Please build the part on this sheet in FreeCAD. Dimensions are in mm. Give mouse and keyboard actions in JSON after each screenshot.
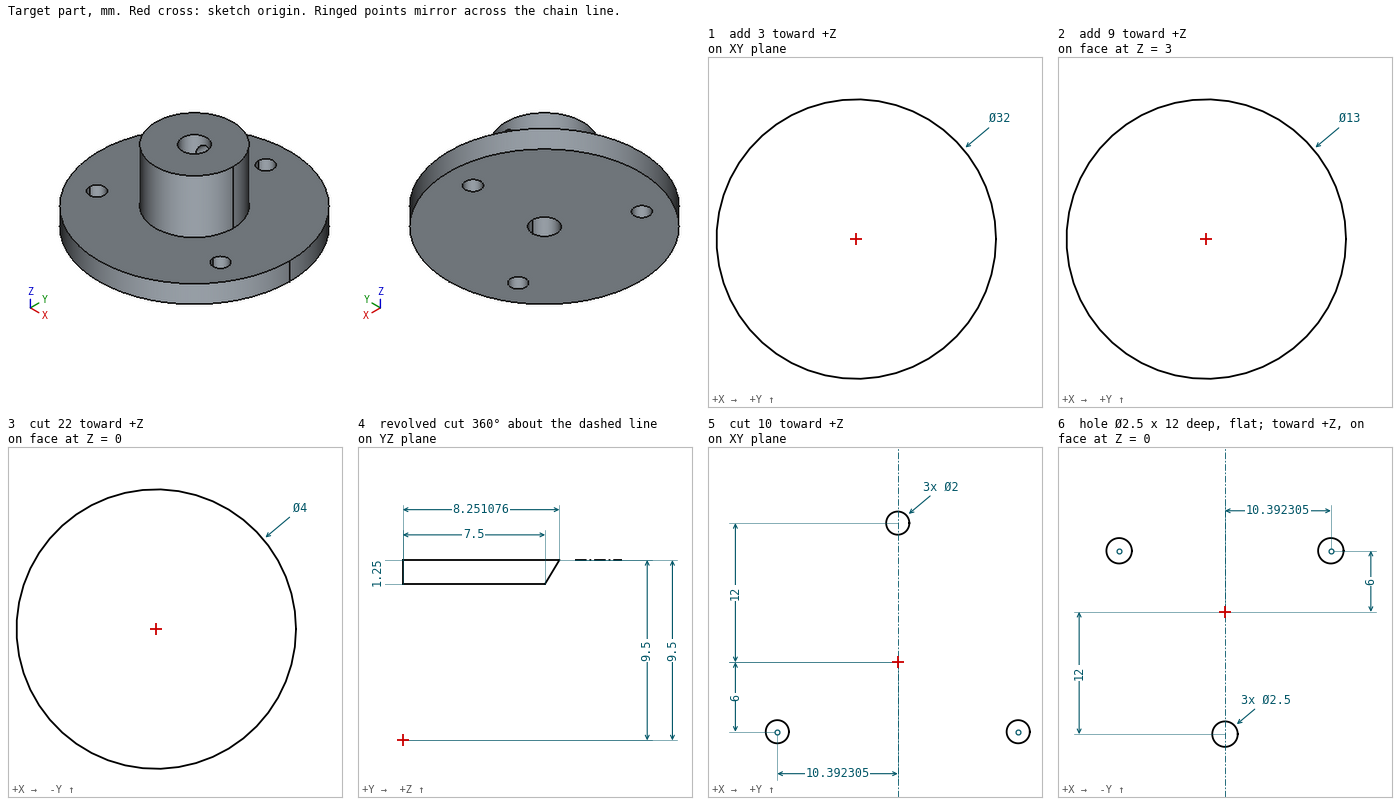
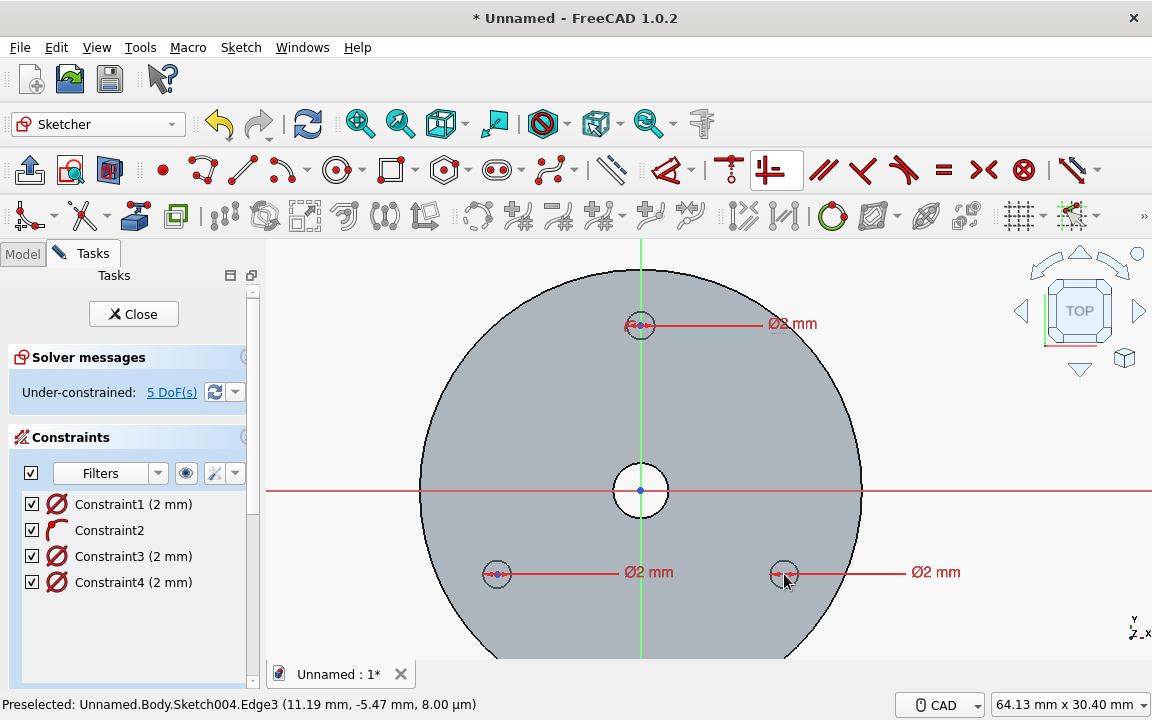
{"action": "left_click", "coordinate": [497, 574]}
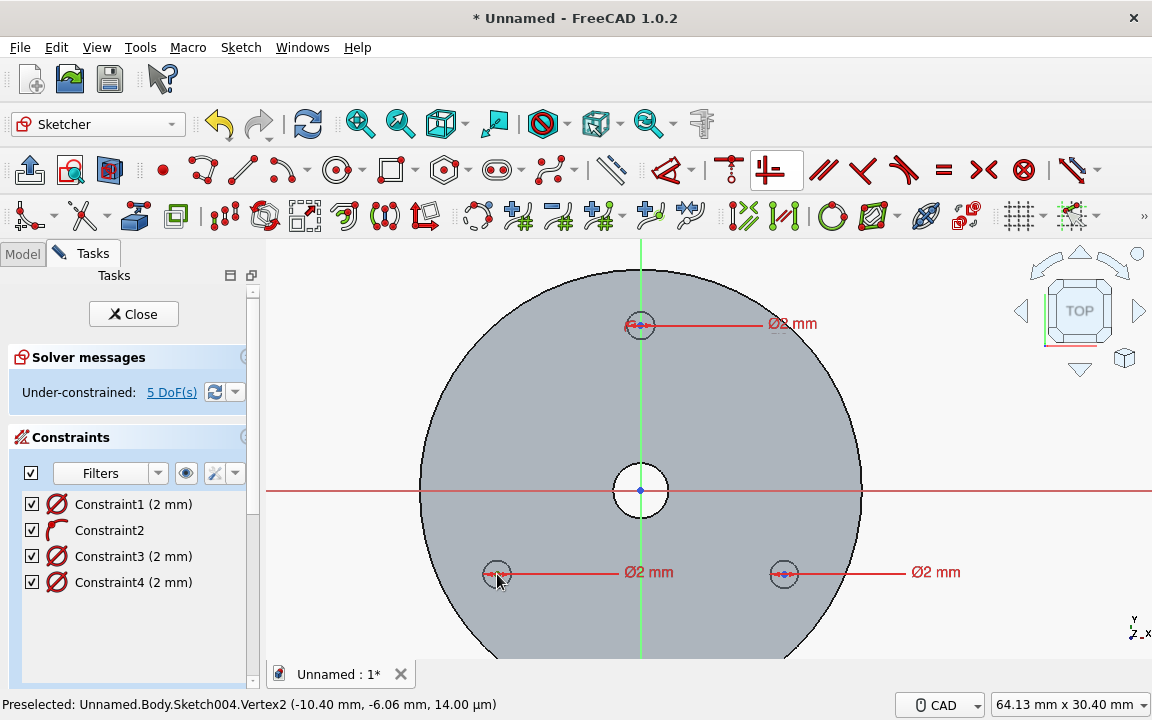
{"action": "left_click", "coordinate": [784, 574]}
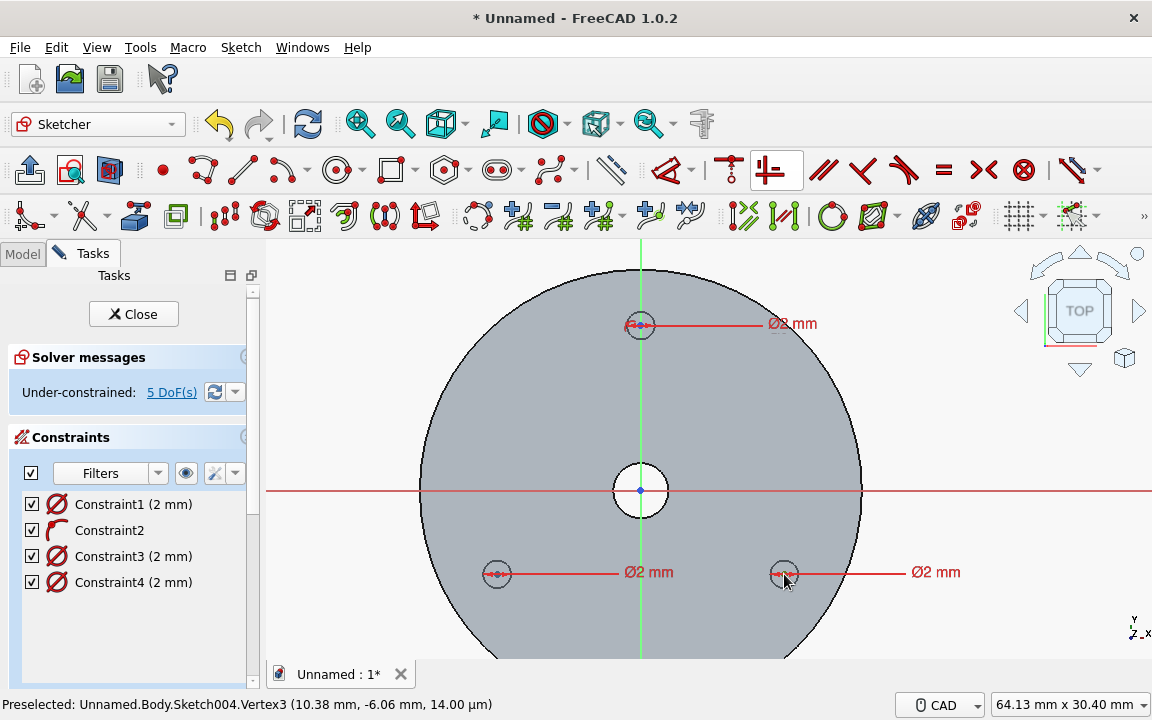
{"action": "left_click", "coordinate": [641, 605]}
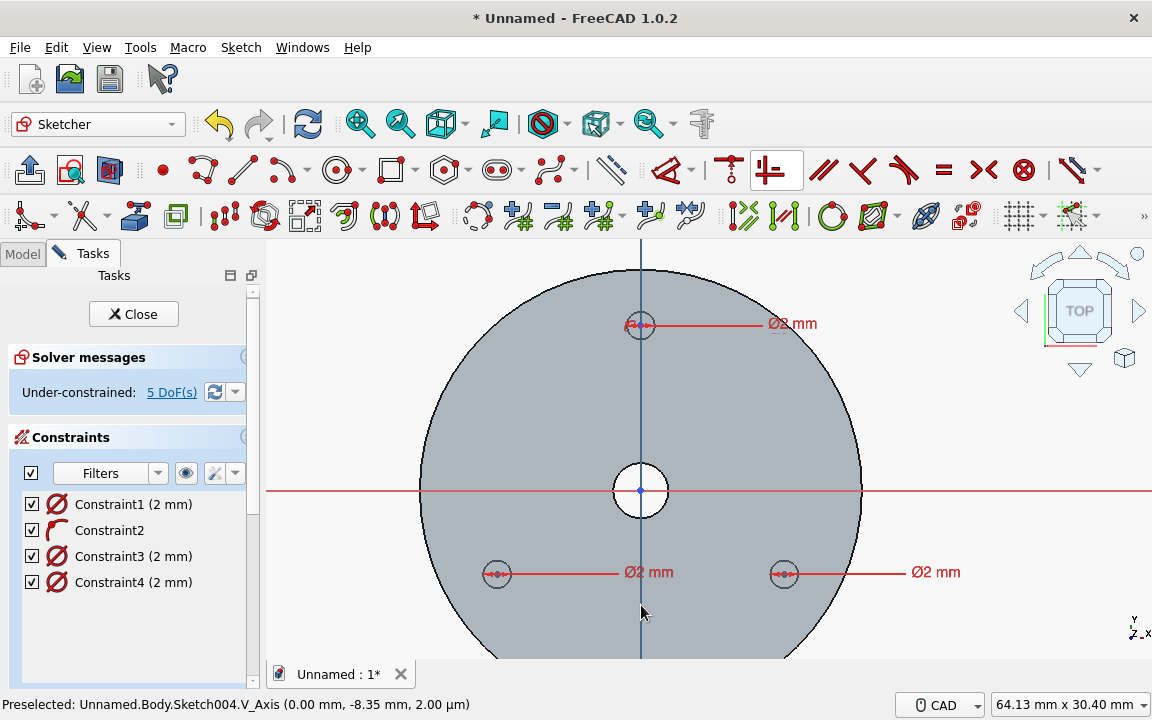
{"action": "left_click", "coordinate": [984, 170]}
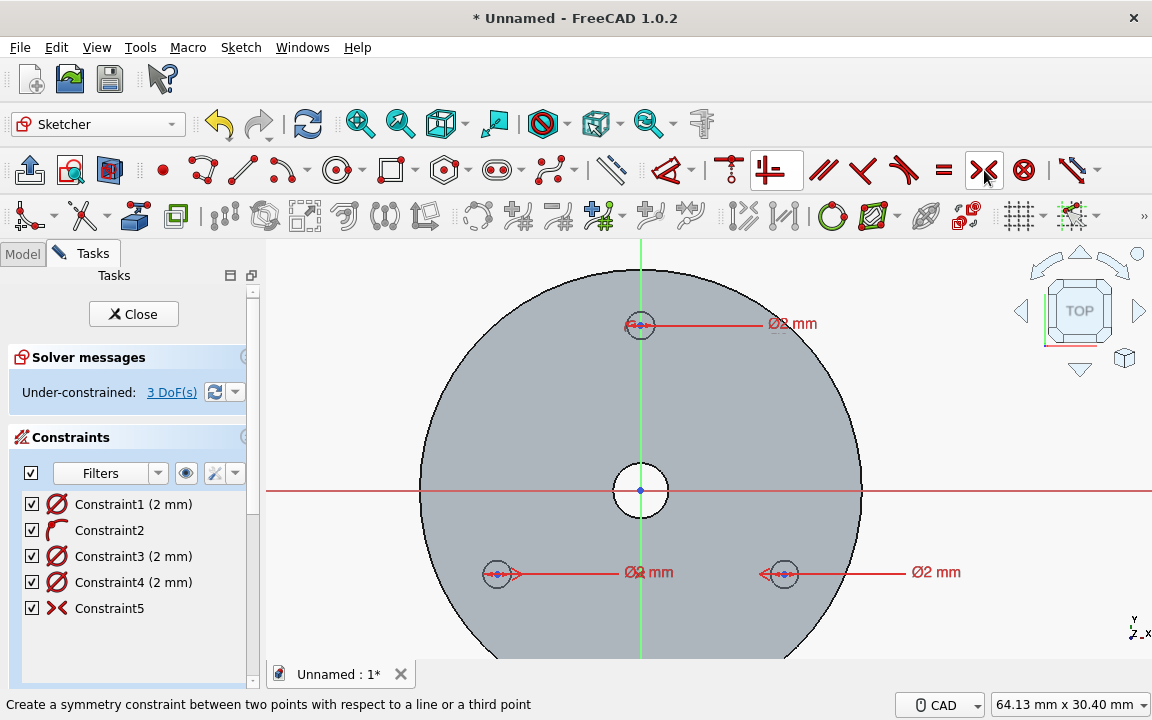
{"action": "left_click", "coordinate": [666, 170]}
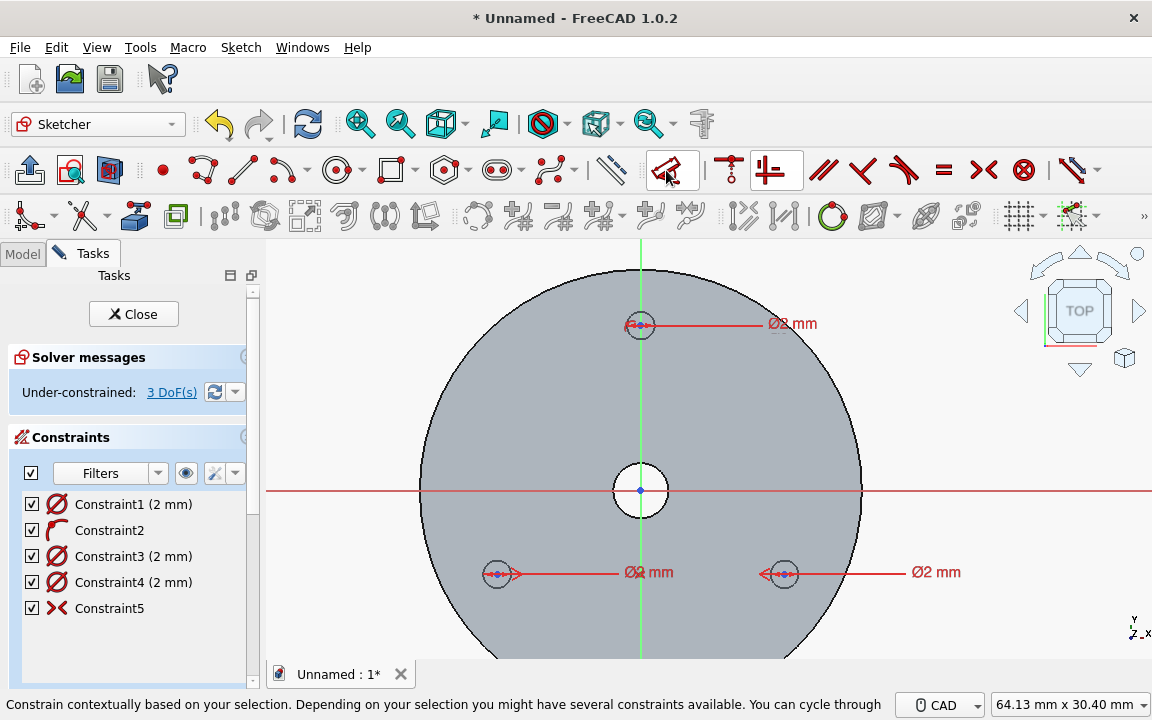
{"action": "left_click", "coordinate": [497, 574]}
{"action": "left_click", "coordinate": [463, 533]}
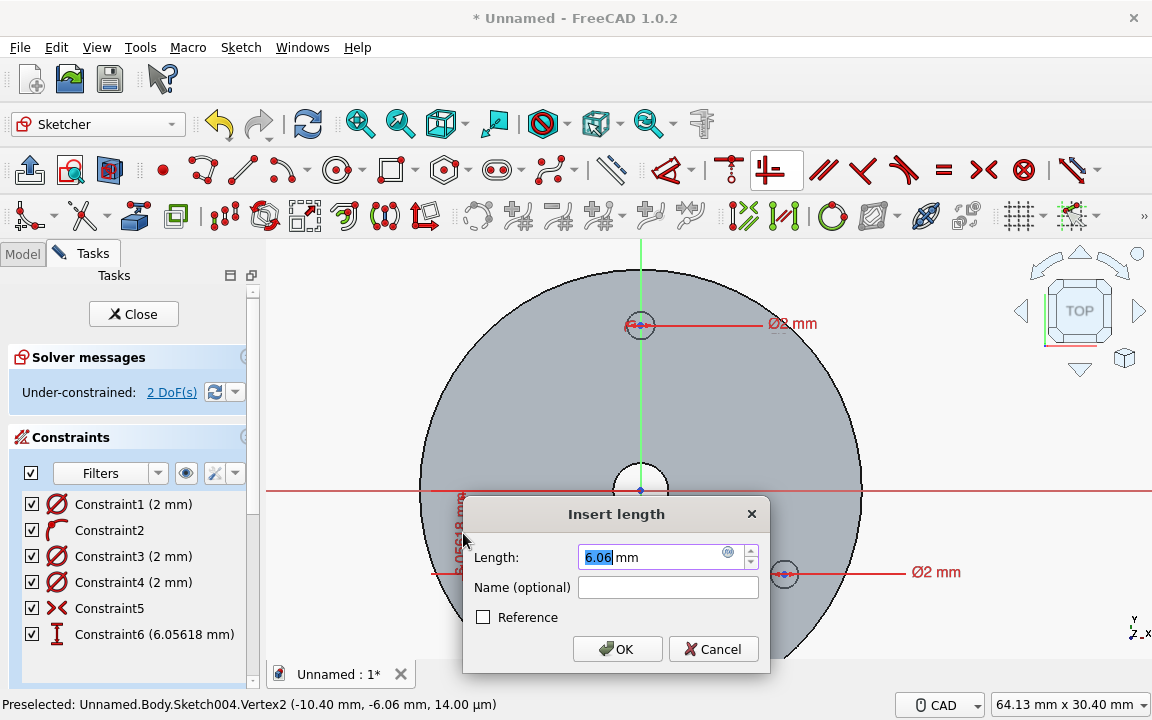
{"action": "type", "text": "6"}
{"action": "key", "text": "Return"}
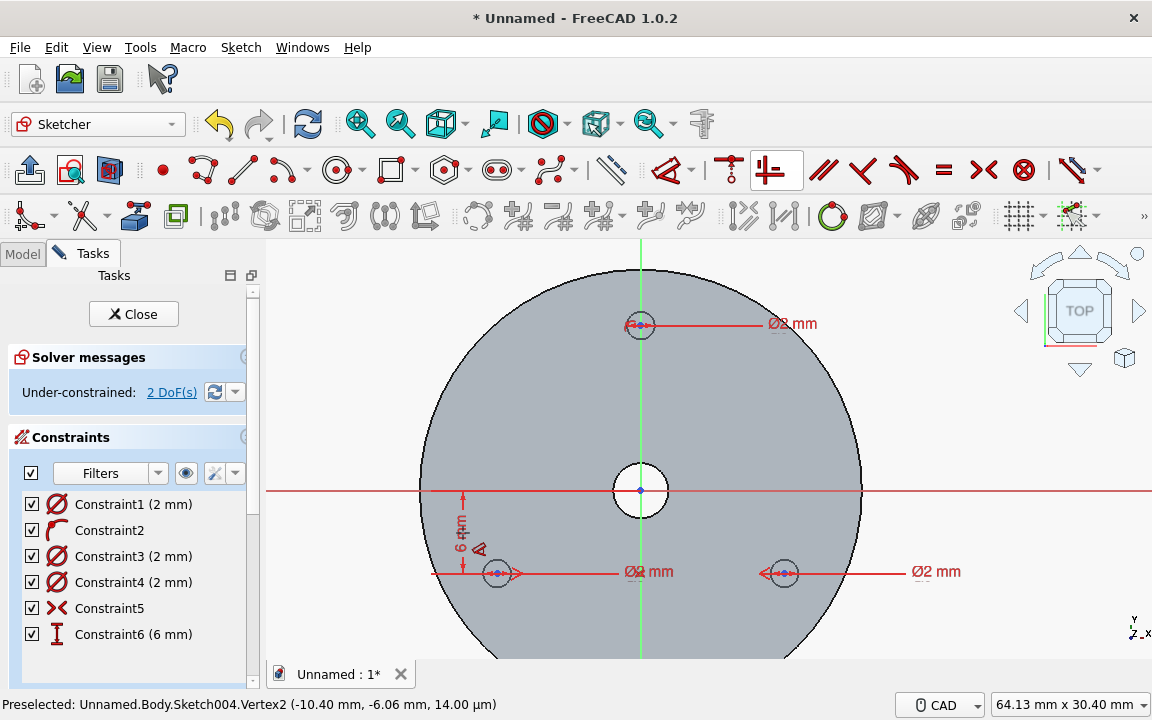
{"action": "left_click", "coordinate": [641, 326]}
{"action": "left_click", "coordinate": [675, 408]}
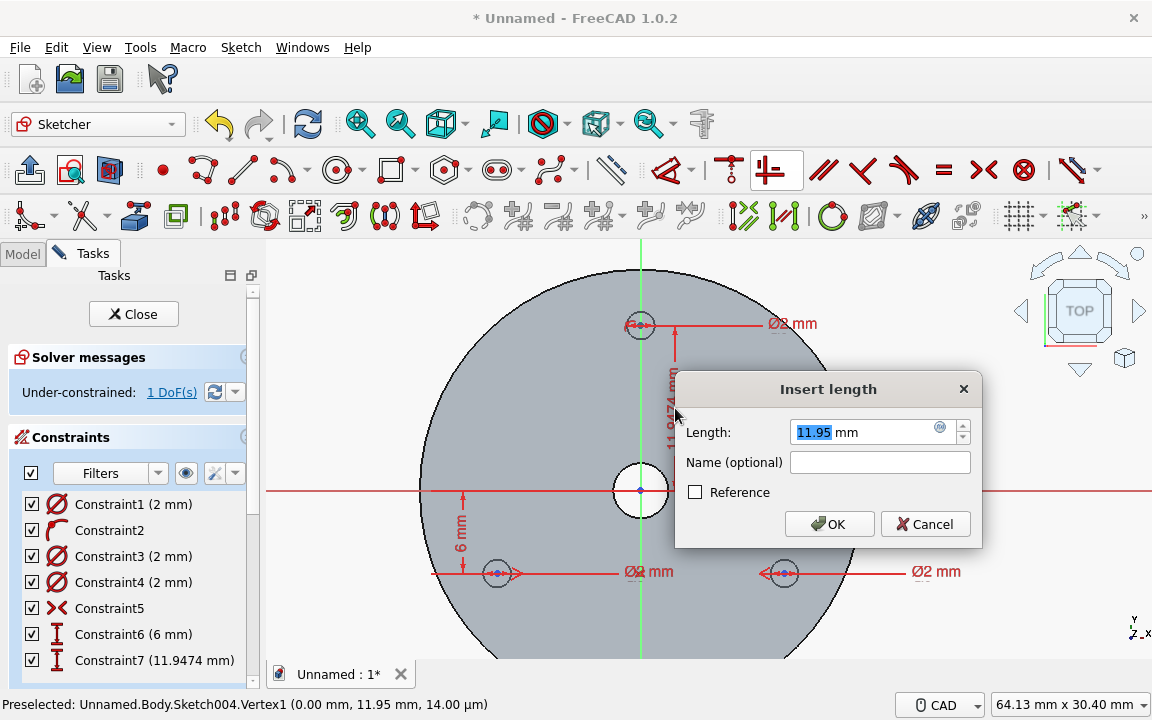
{"action": "type", "text": "12"}
{"action": "key", "text": "Return"}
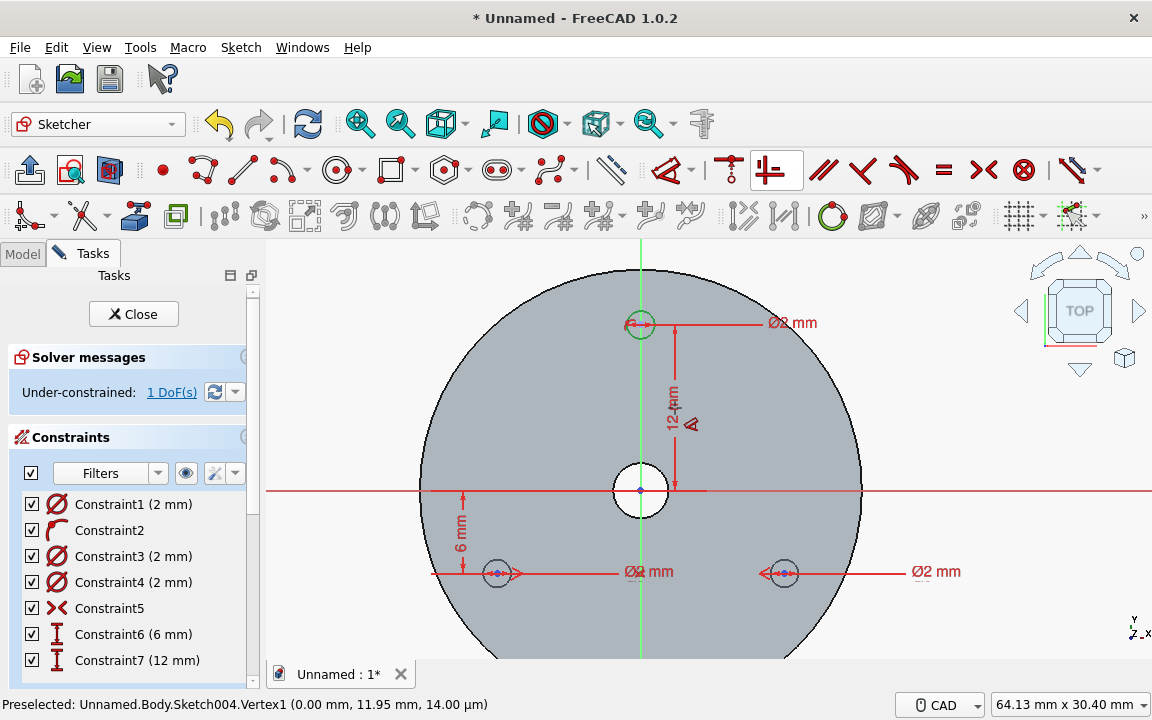
{"action": "left_click", "coordinate": [497, 574]}
{"action": "left_click", "coordinate": [569, 608]}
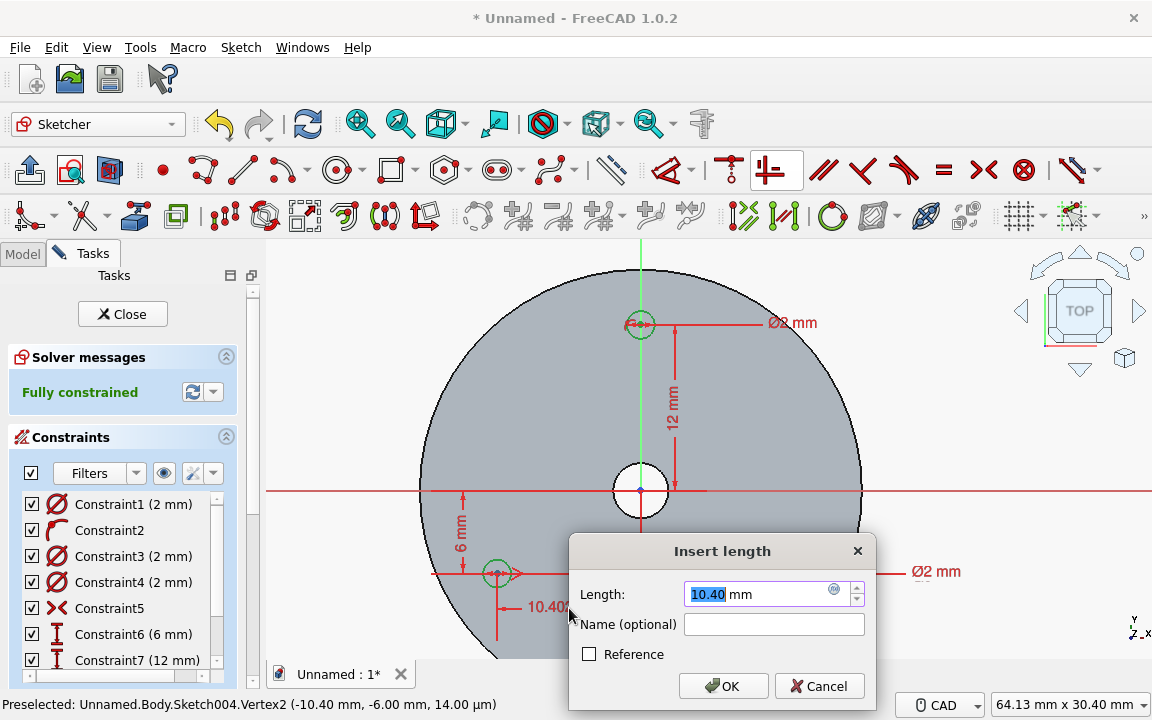
{"action": "type", "text": "10.392305"}
{"action": "key", "text": "Return"}
{"action": "key", "text": "Escape"}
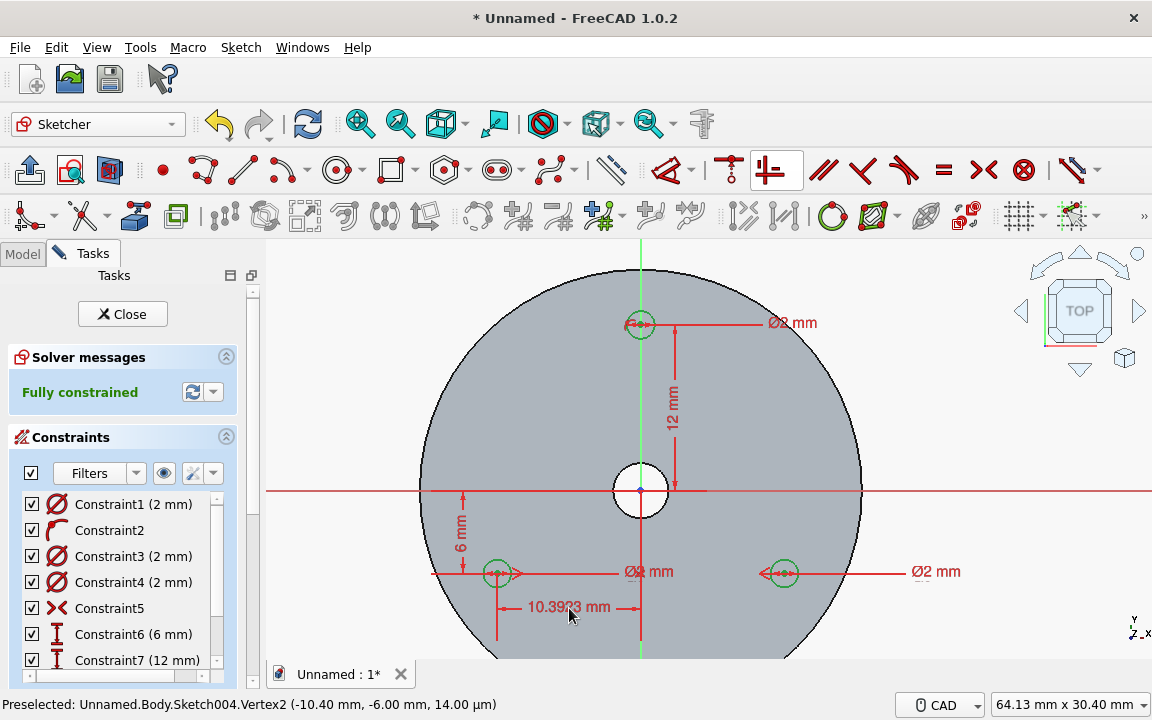
{"action": "left_click", "coordinate": [123, 314]}